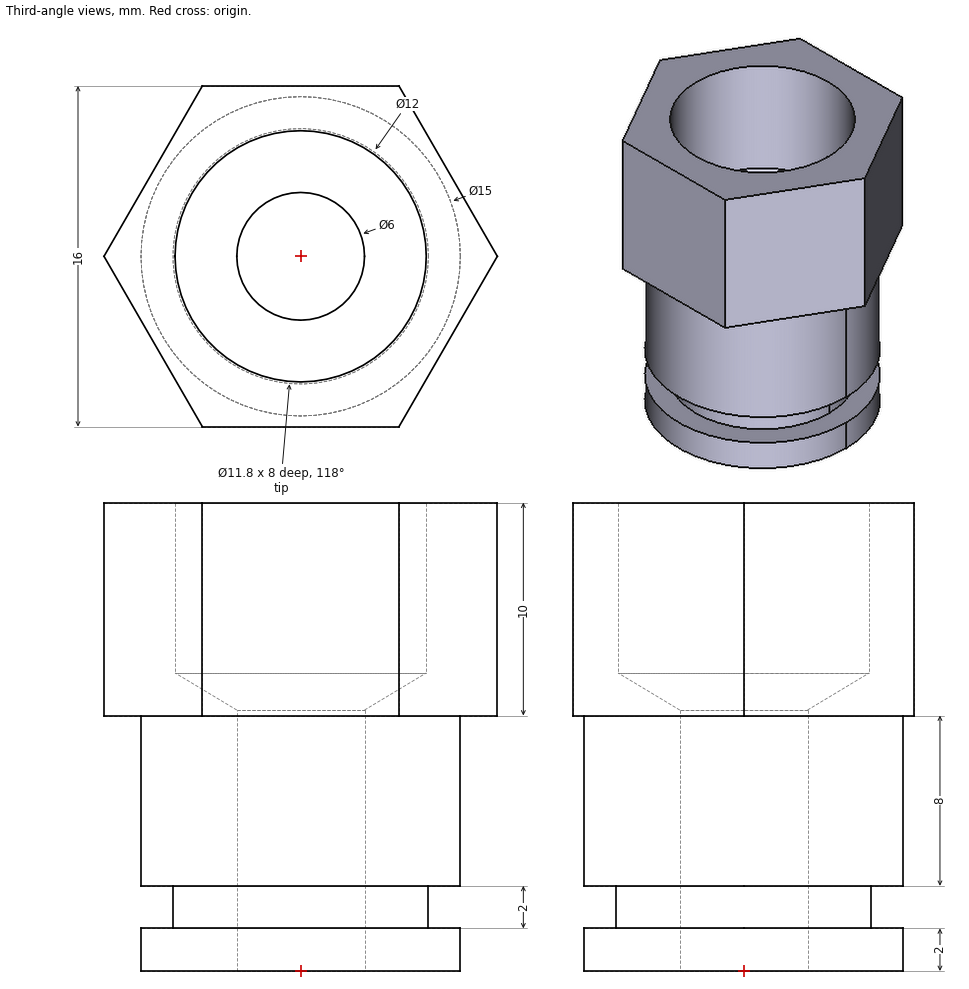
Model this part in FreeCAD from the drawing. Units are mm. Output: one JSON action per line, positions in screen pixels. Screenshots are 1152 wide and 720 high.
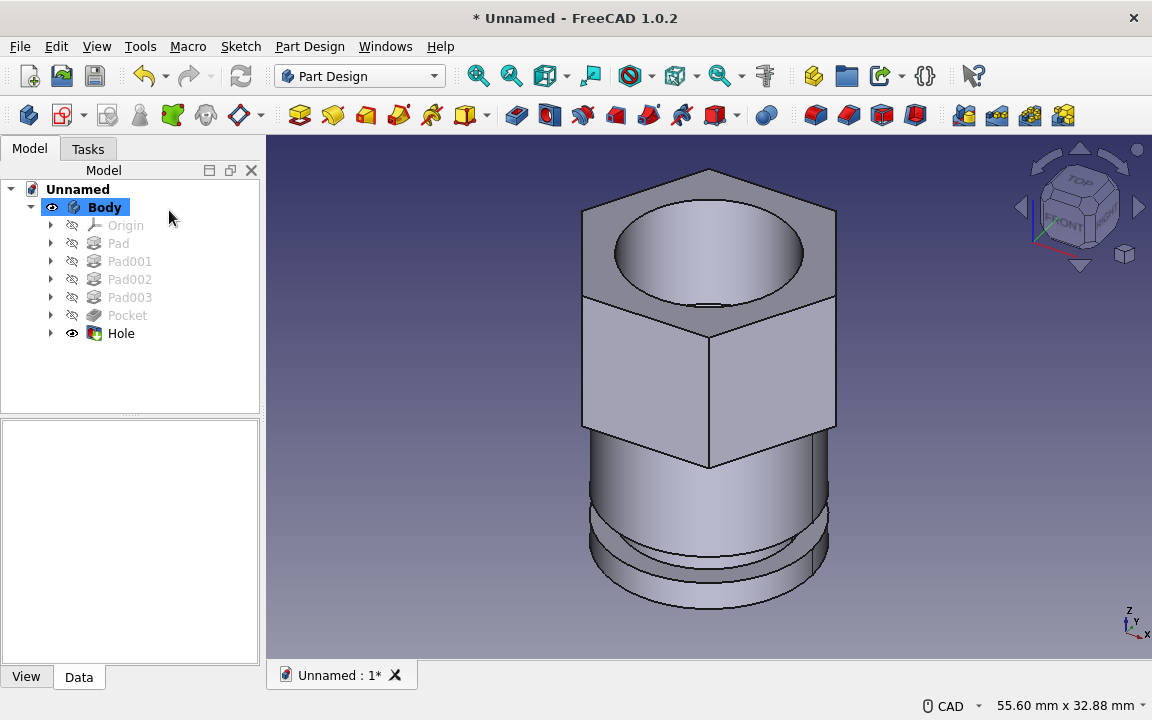
{"action": "key", "text": "0"}